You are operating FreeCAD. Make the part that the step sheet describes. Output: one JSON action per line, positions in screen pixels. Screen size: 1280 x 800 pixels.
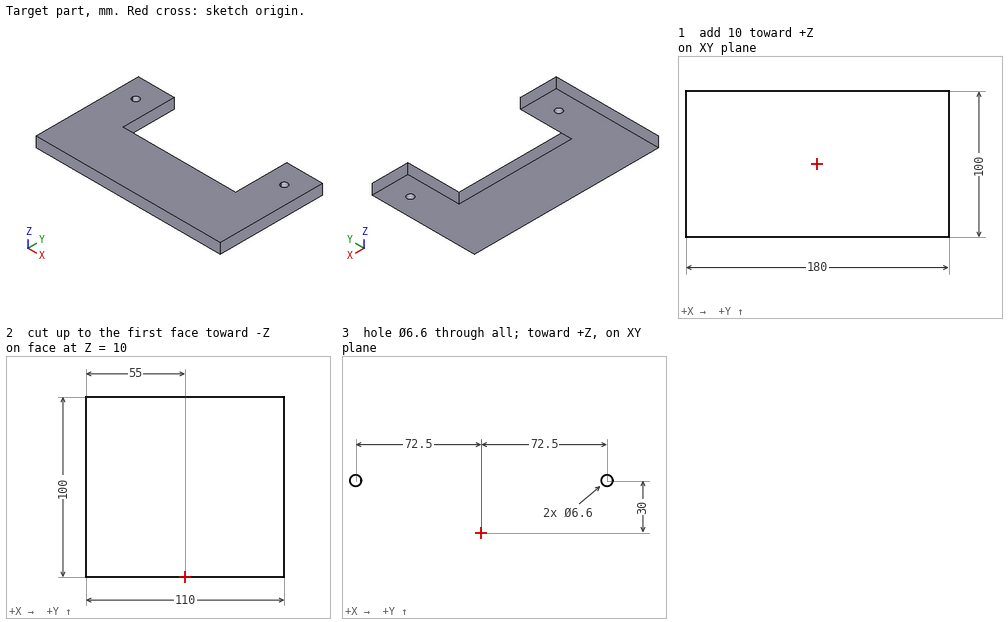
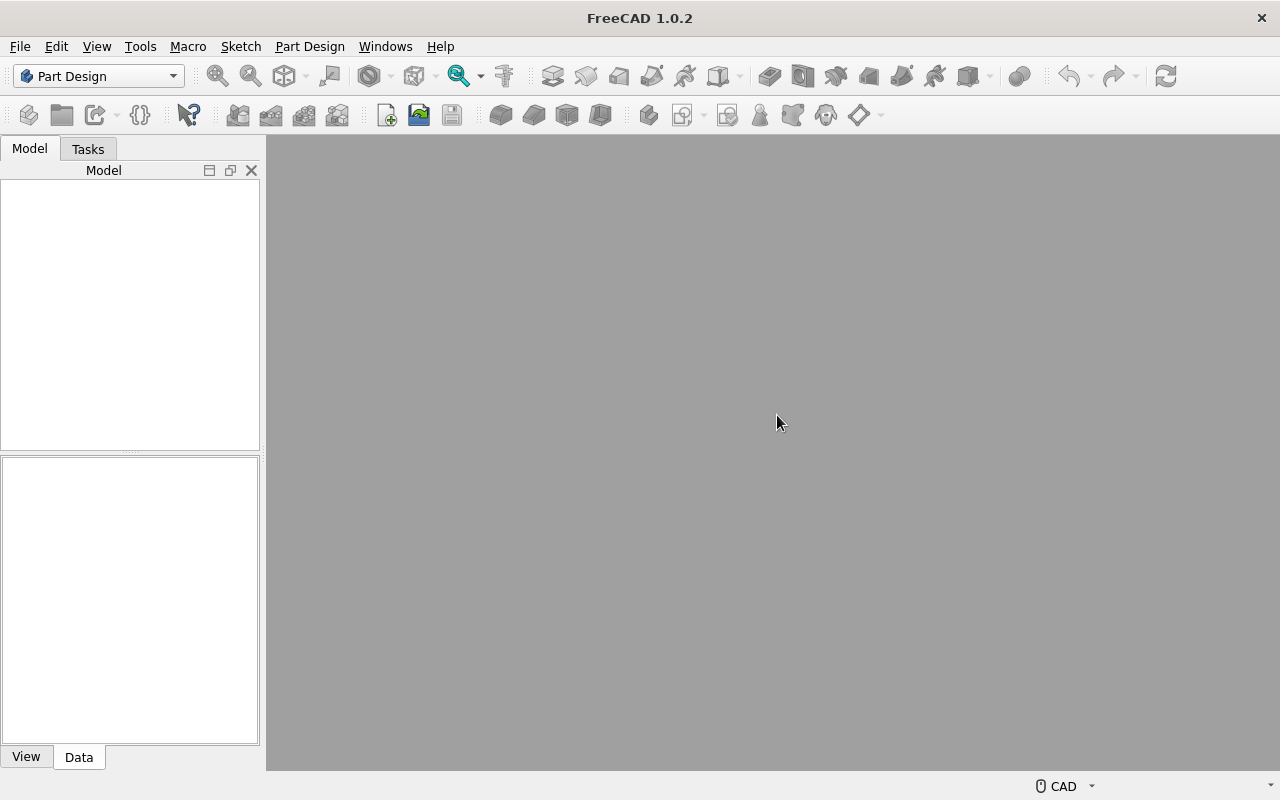
{"action": "left_click", "coordinate": [386, 116]}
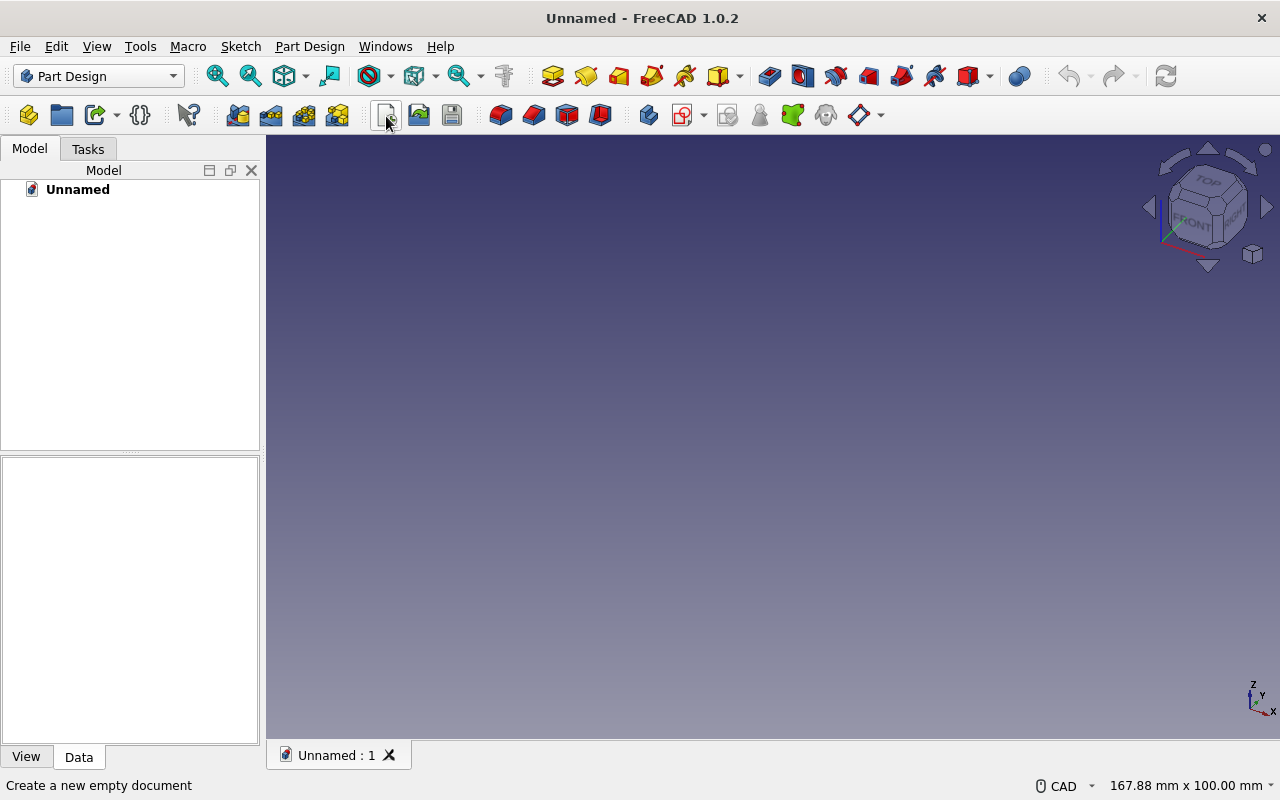
{"action": "left_click", "coordinate": [682, 116]}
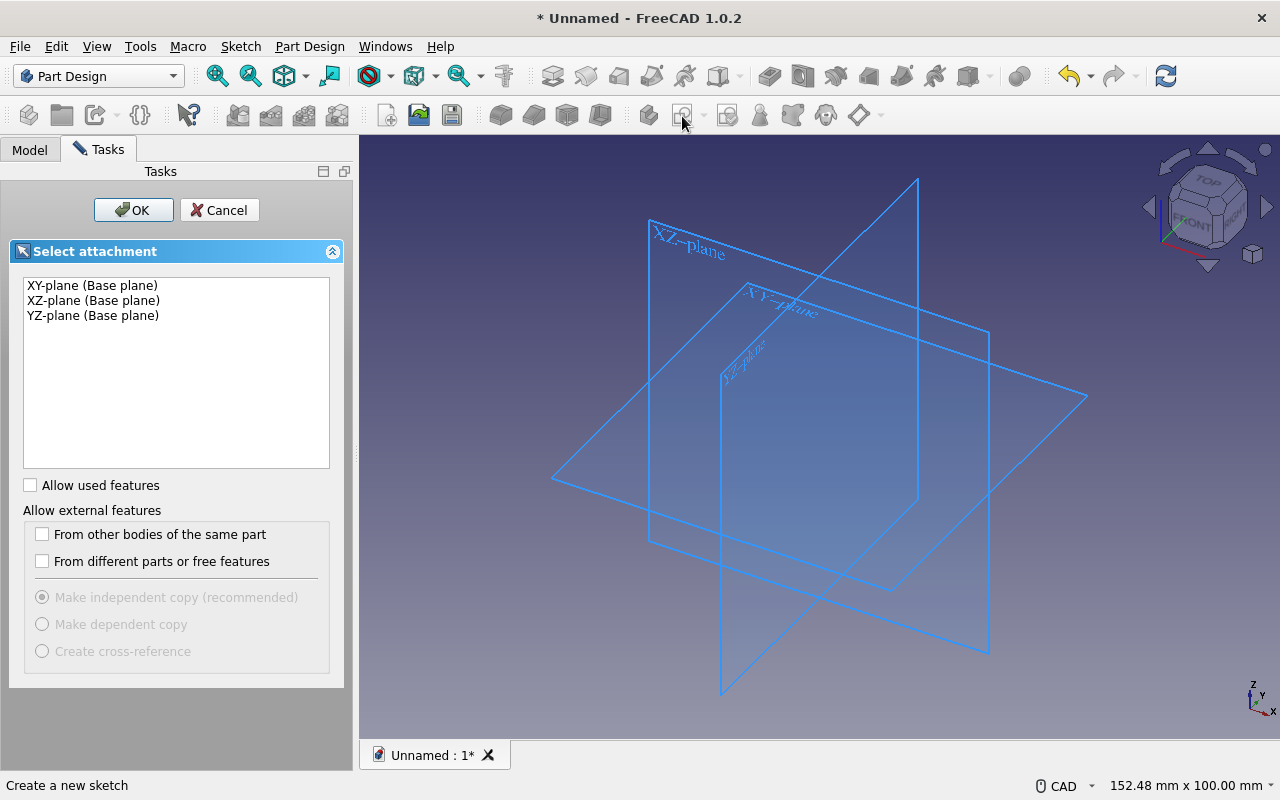
{"action": "left_click", "coordinate": [84, 286]}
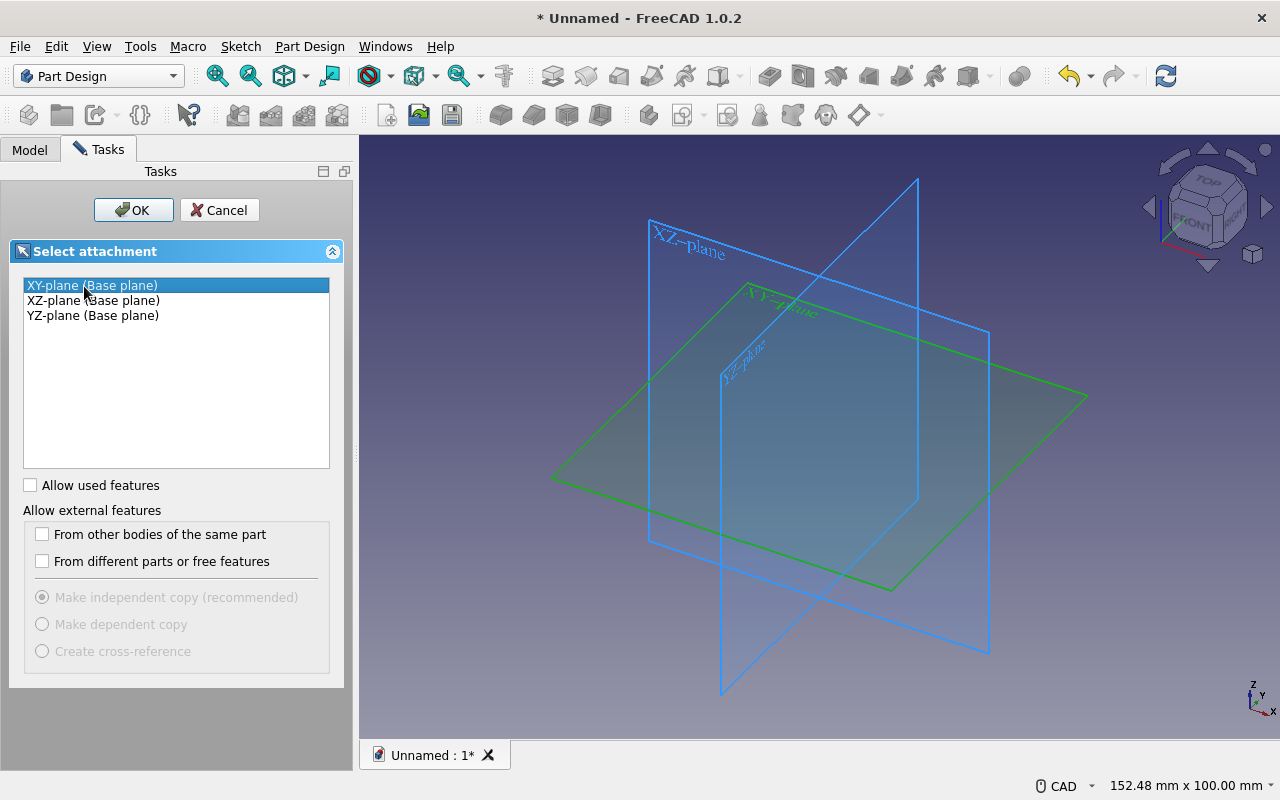
{"action": "left_click", "coordinate": [134, 210]}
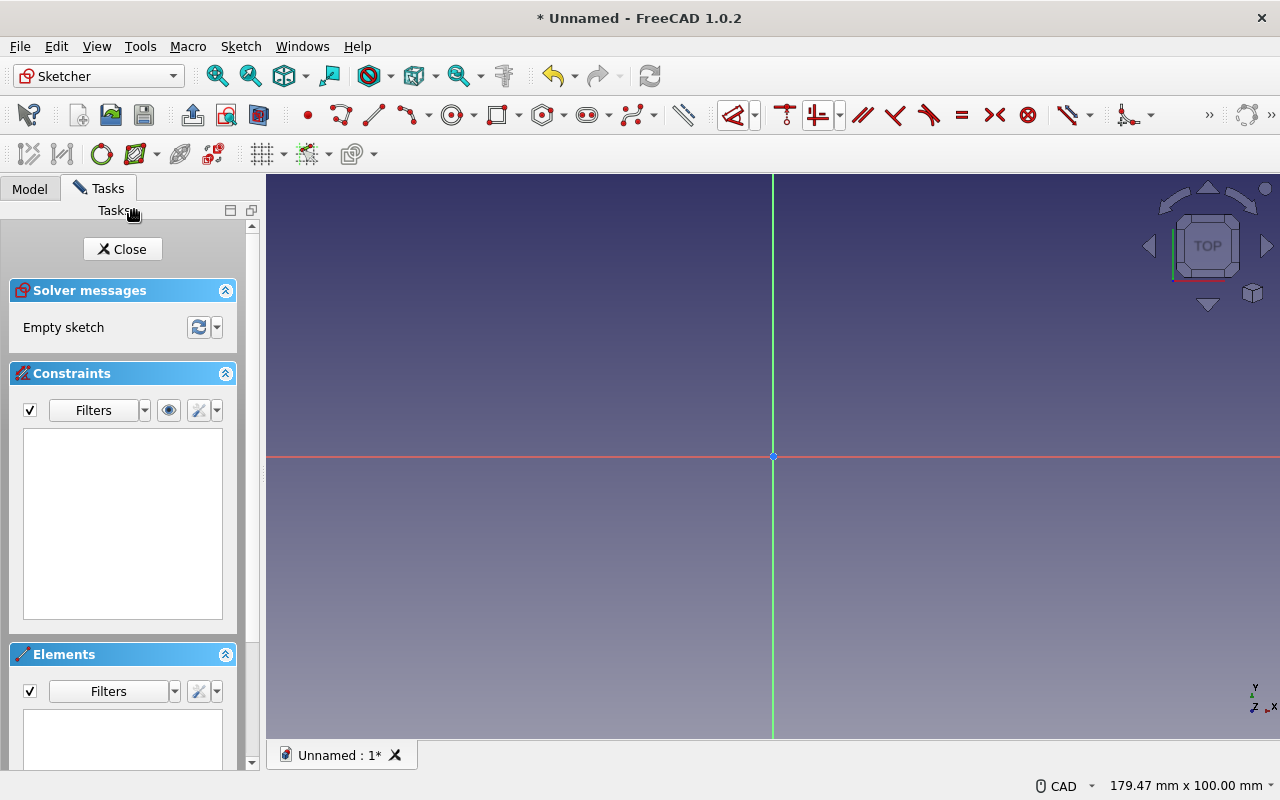
{"action": "scroll", "coordinate": [621, 456], "scroll_direction": "down", "scroll_amount": 3}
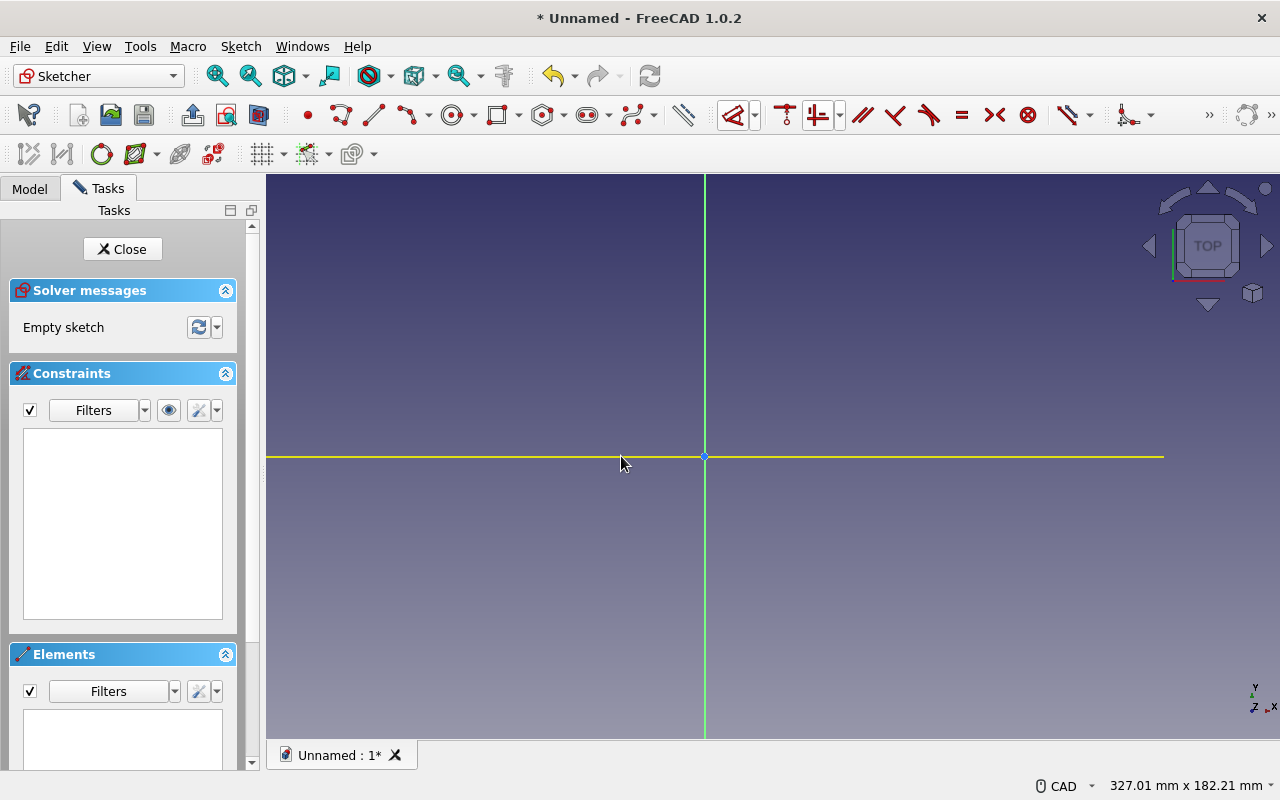
{"action": "left_click", "coordinate": [518, 116]}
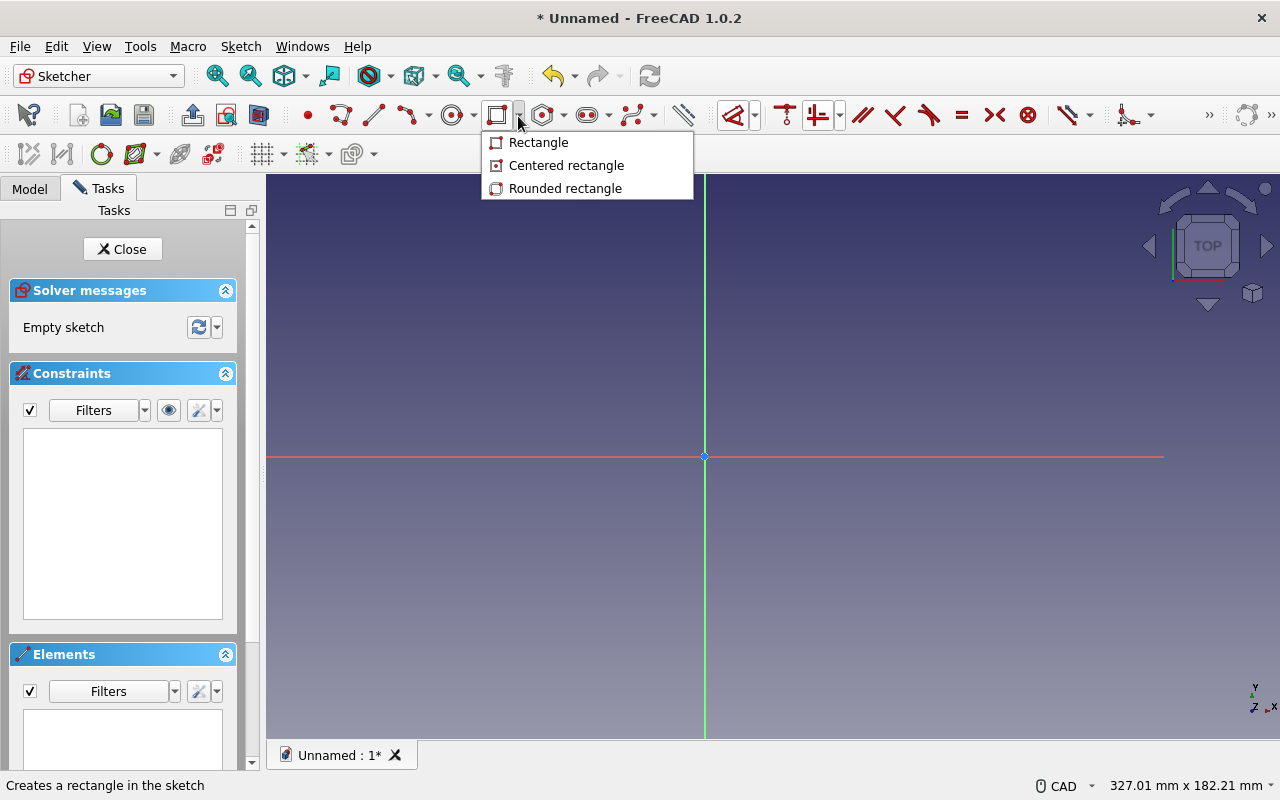
{"action": "left_click", "coordinate": [588, 166]}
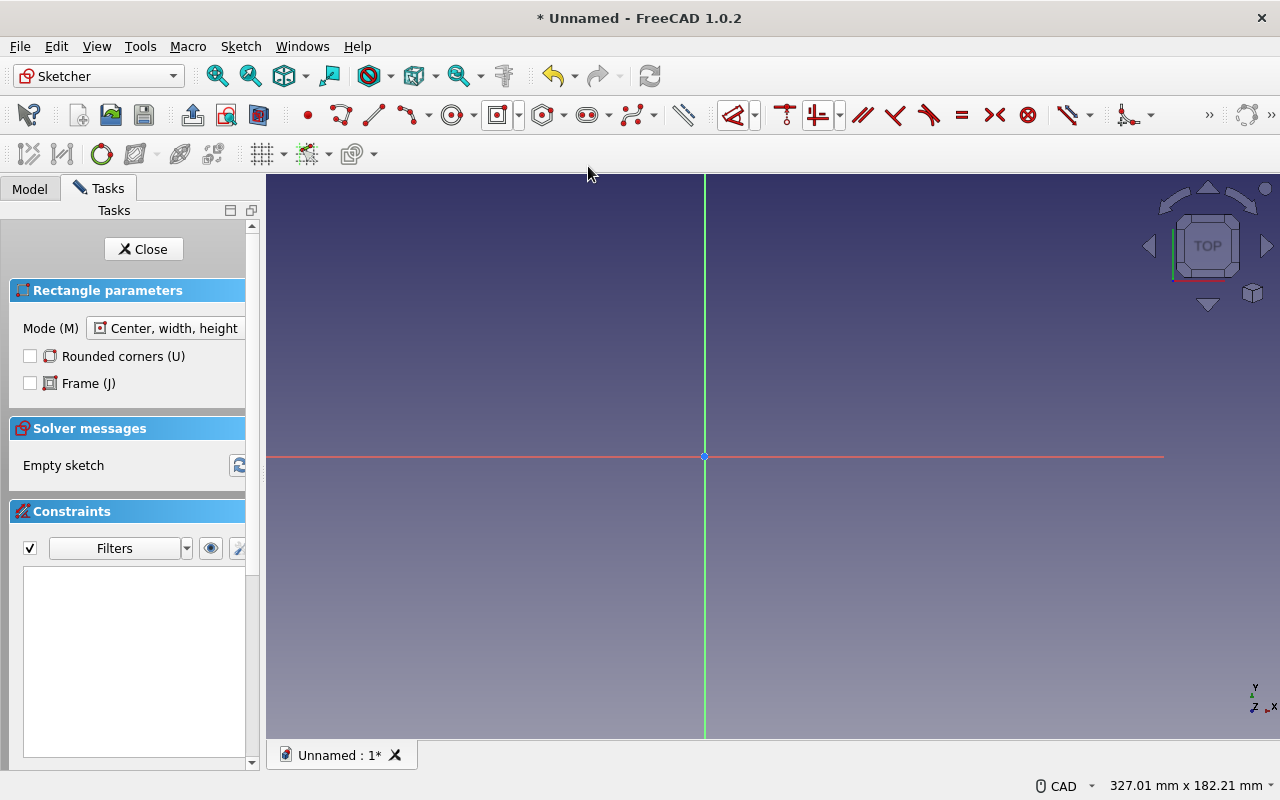
{"action": "left_click", "coordinate": [705, 456]}
{"action": "left_click", "coordinate": [984, 301]}
{"action": "key", "text": "Escape"}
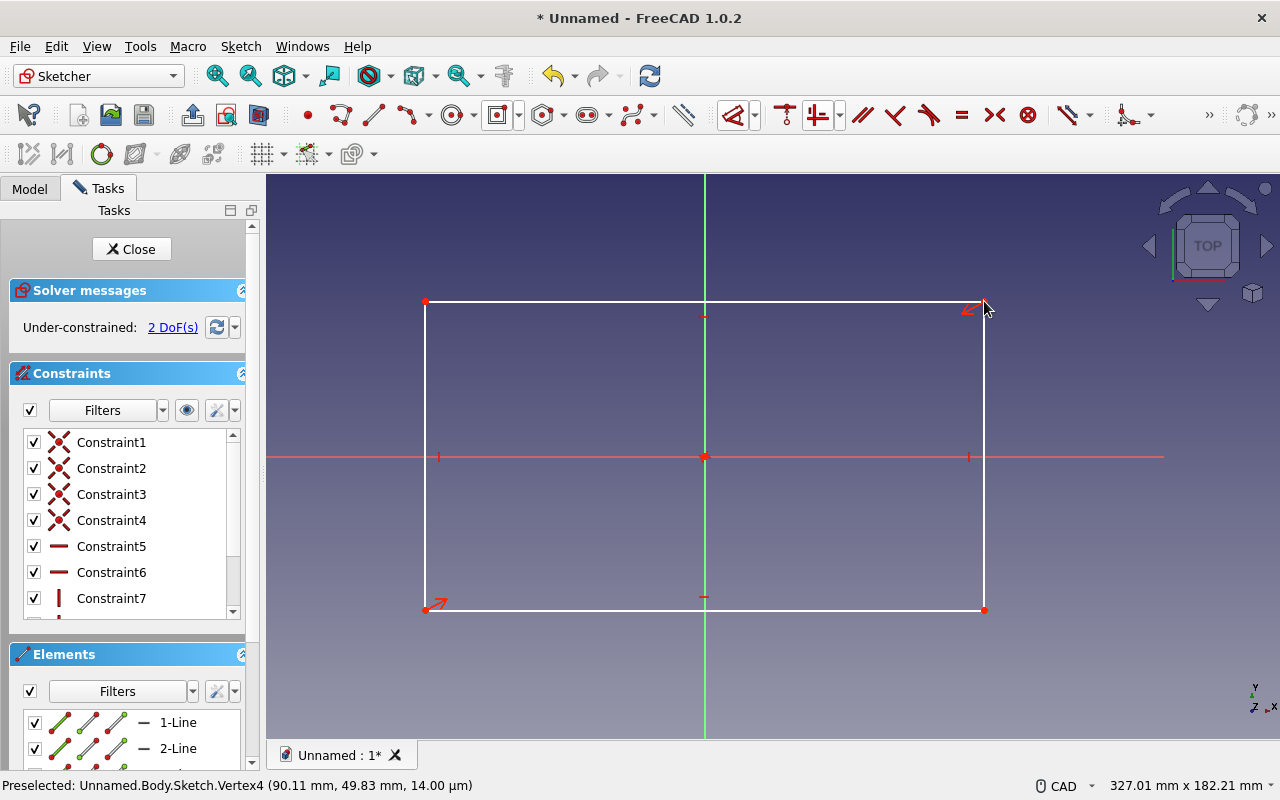
{"action": "left_click", "coordinate": [593, 611]}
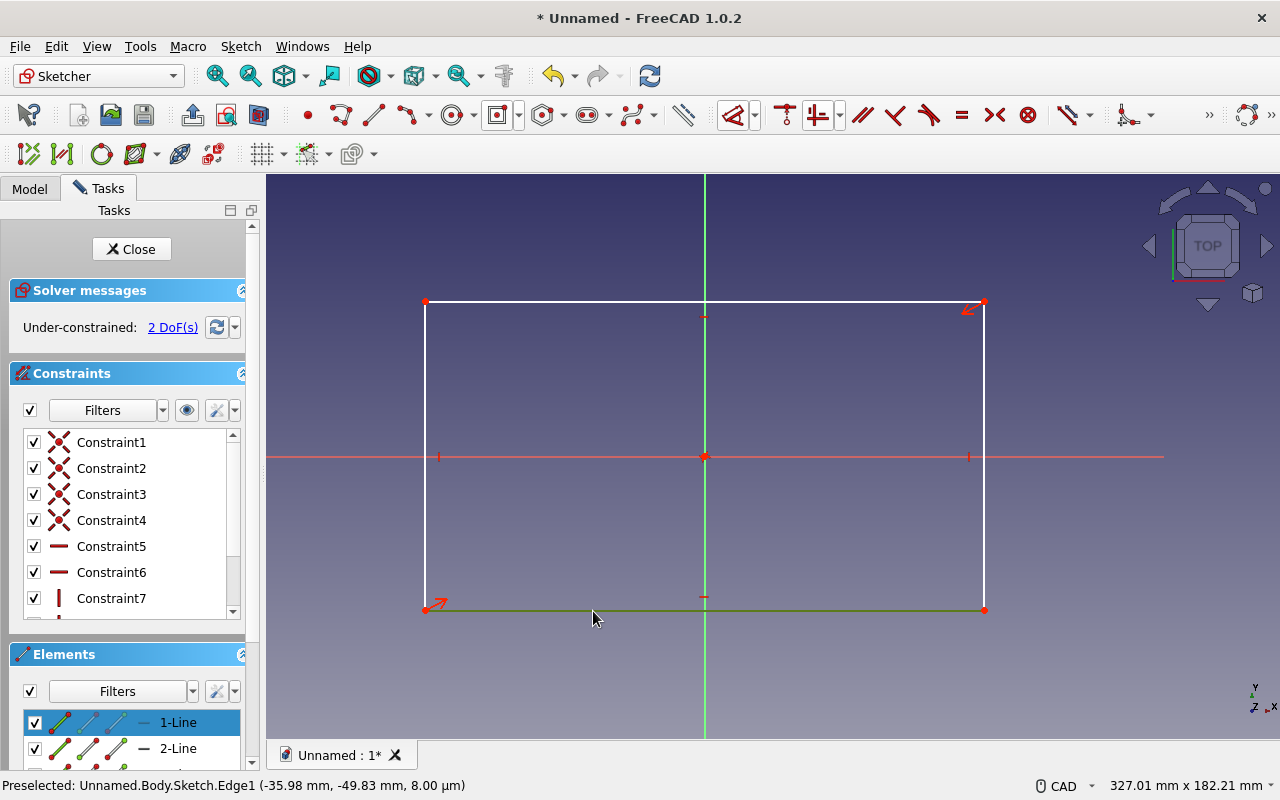
{"action": "key", "text": "l"}